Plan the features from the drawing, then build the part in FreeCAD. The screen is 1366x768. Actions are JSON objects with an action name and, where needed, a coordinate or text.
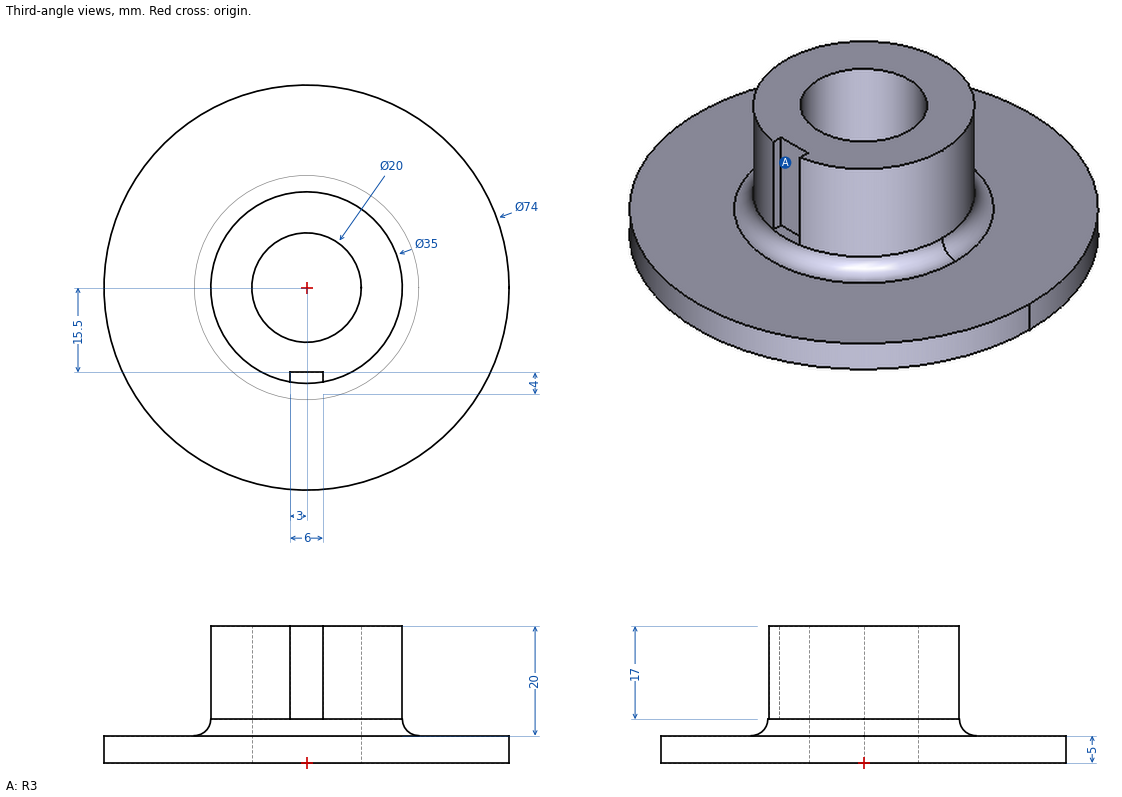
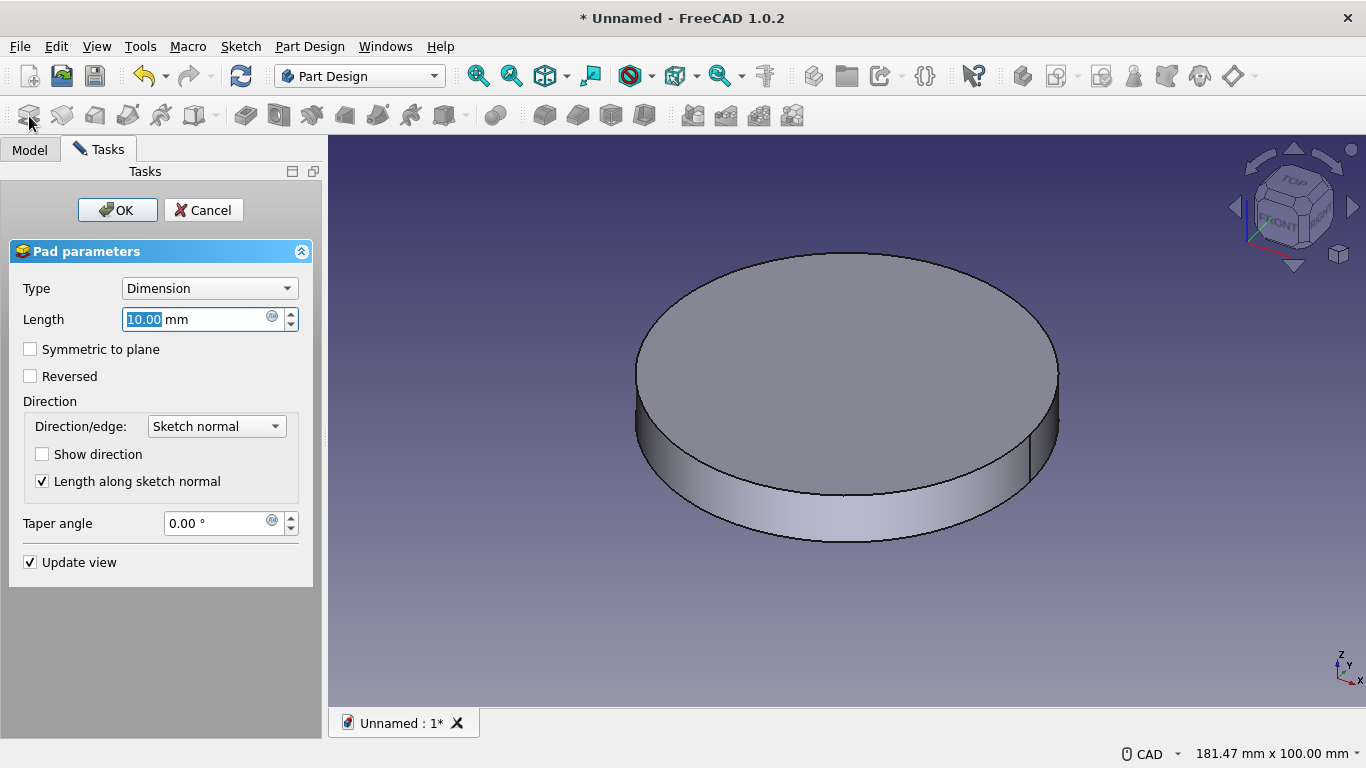
{"action": "type", "text": "5"}
{"action": "key", "text": "Tab"}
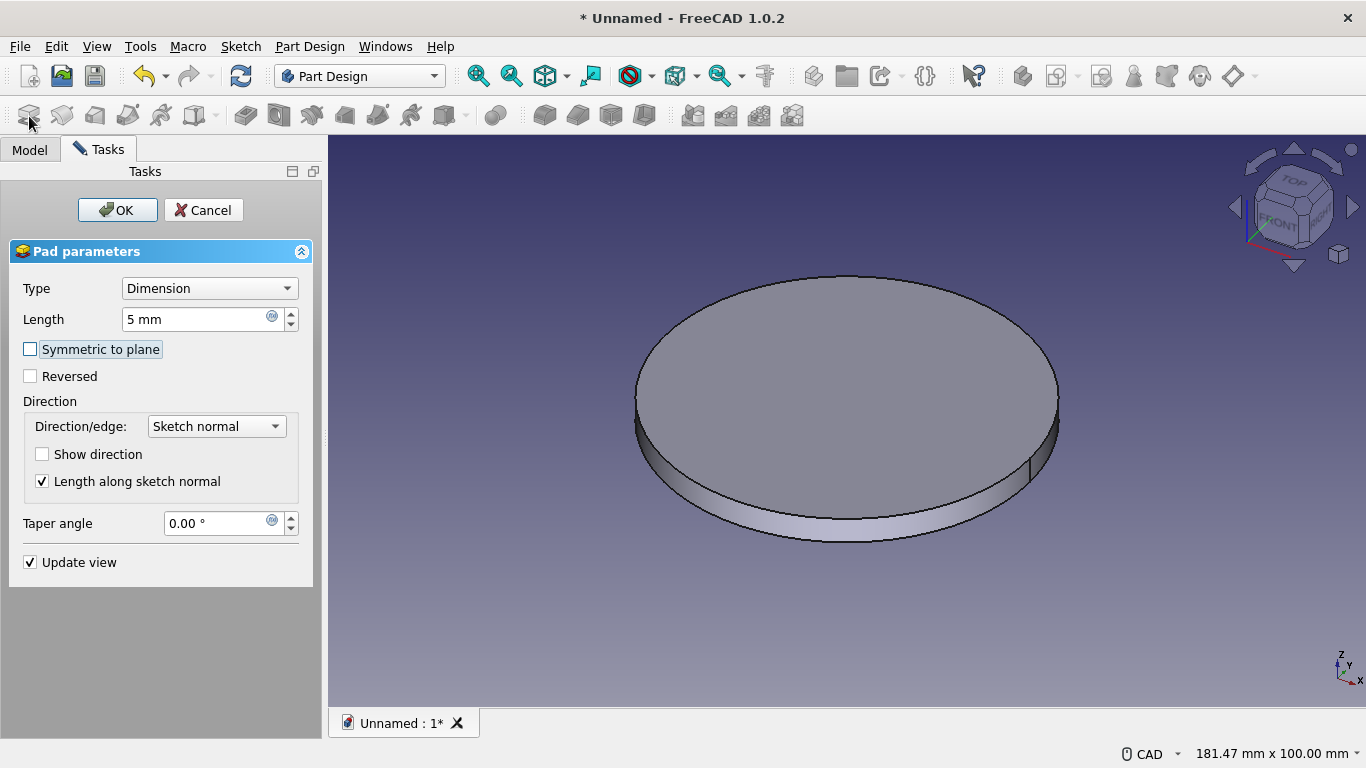
{"action": "left_click", "coordinate": [118, 210]}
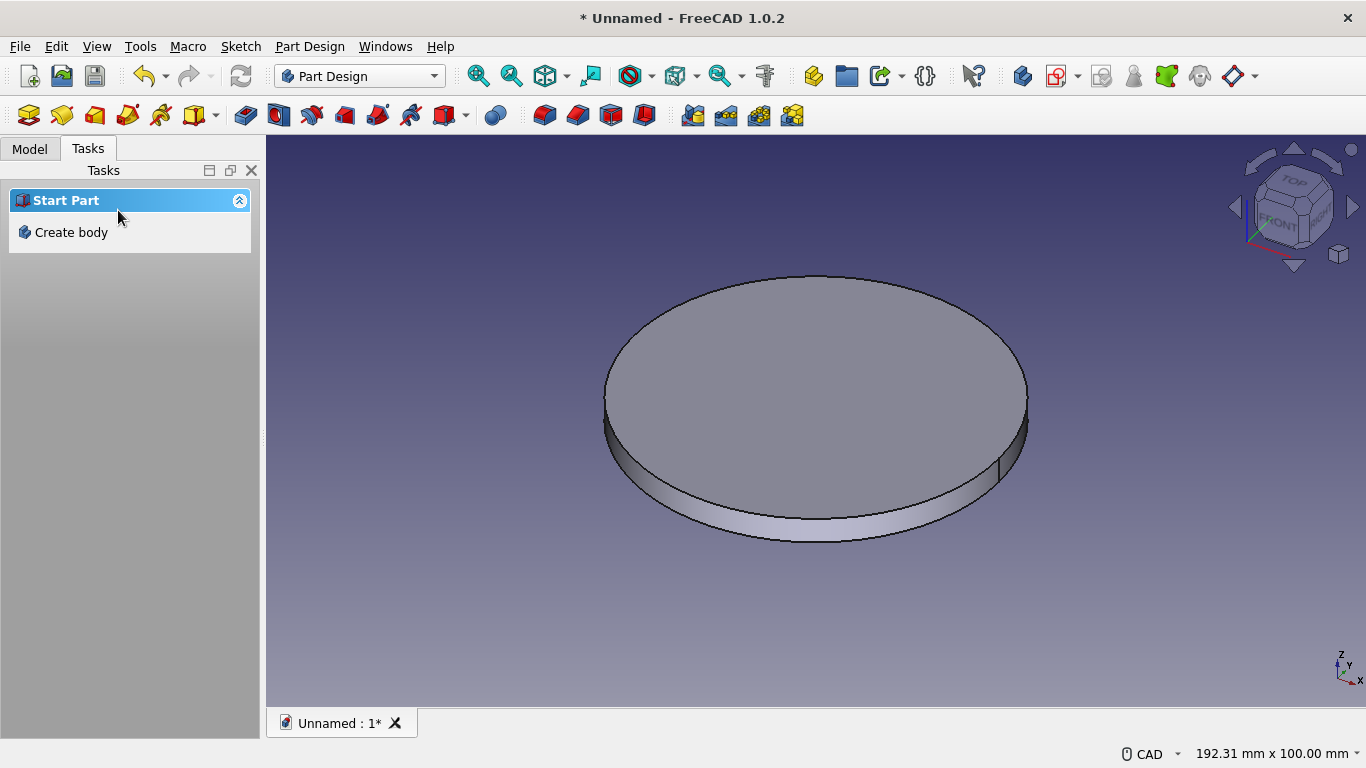
{"action": "left_click", "coordinate": [816, 397]}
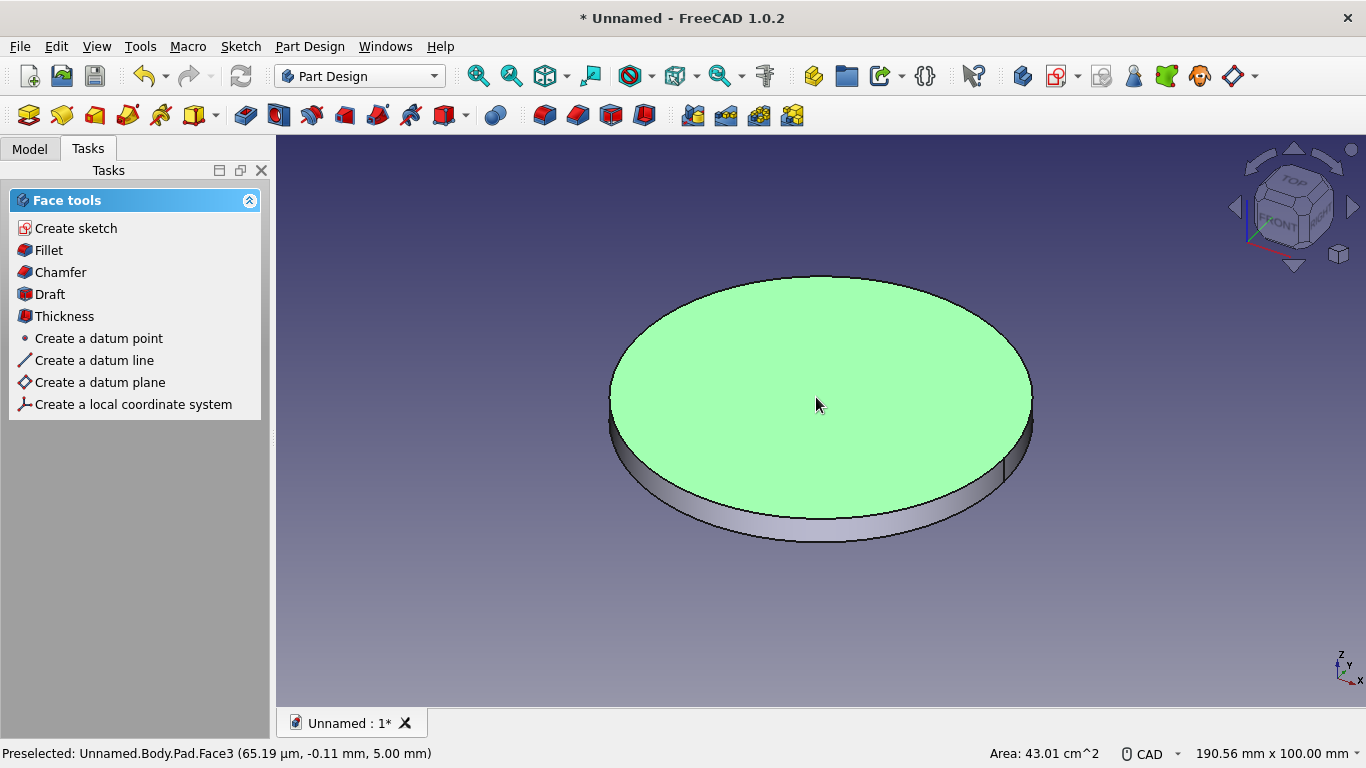
{"action": "left_click", "coordinate": [1056, 76]}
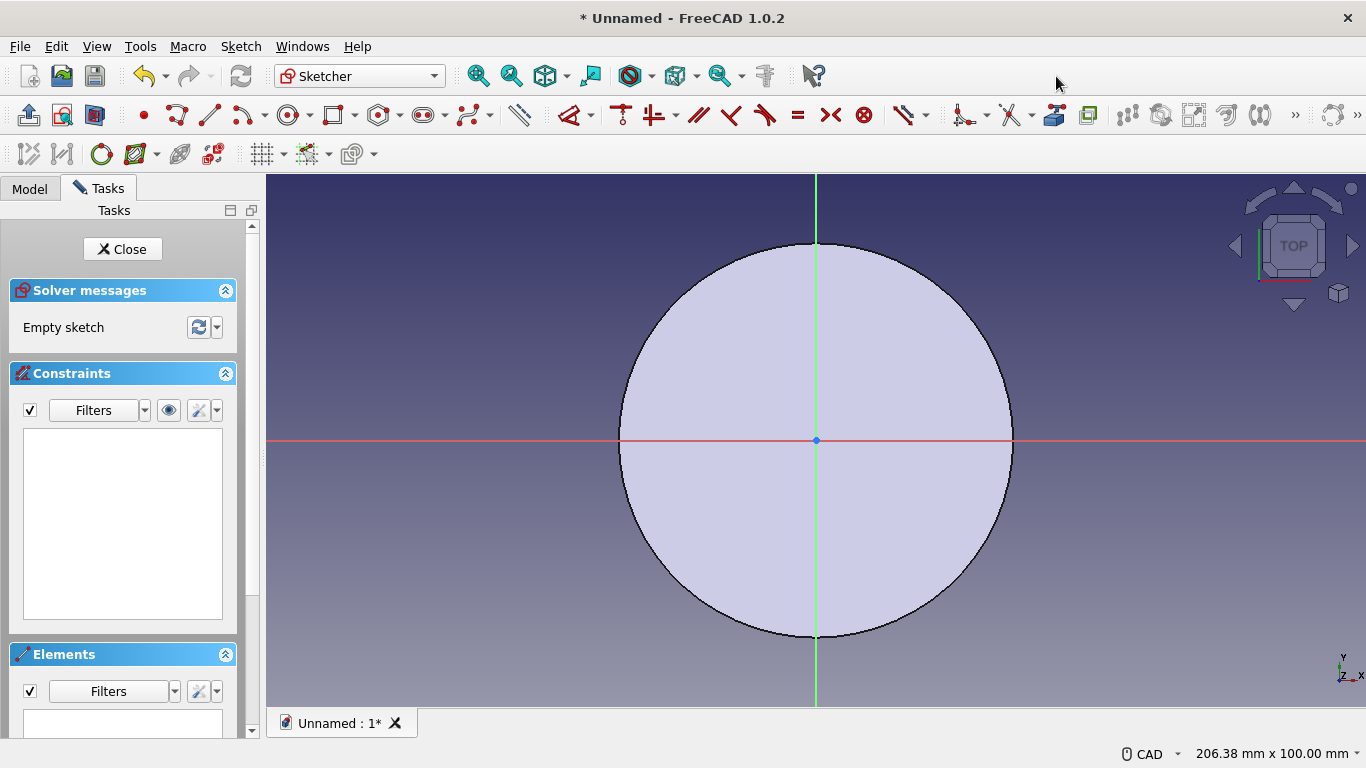
{"action": "scroll", "coordinate": [899, 441], "scroll_direction": "up", "scroll_amount": 3}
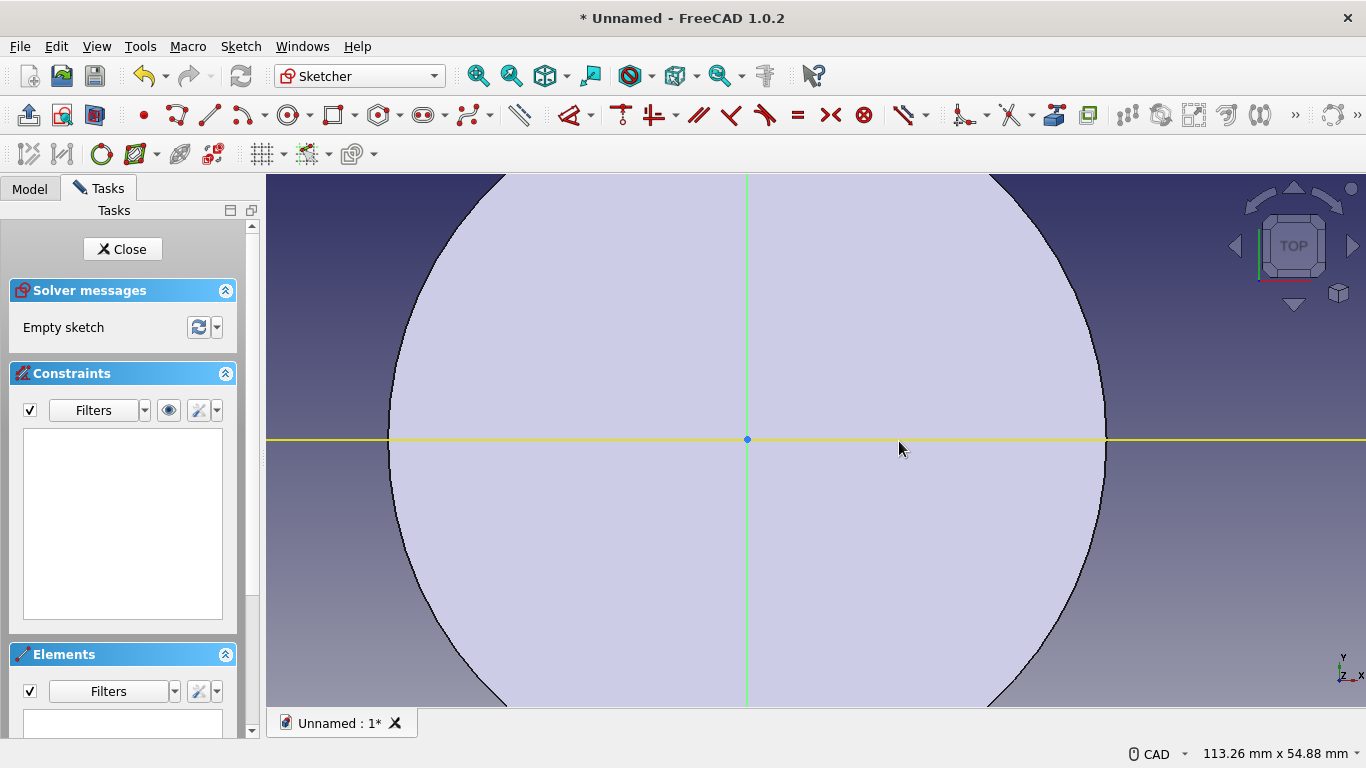
{"action": "left_click", "coordinate": [288, 116]}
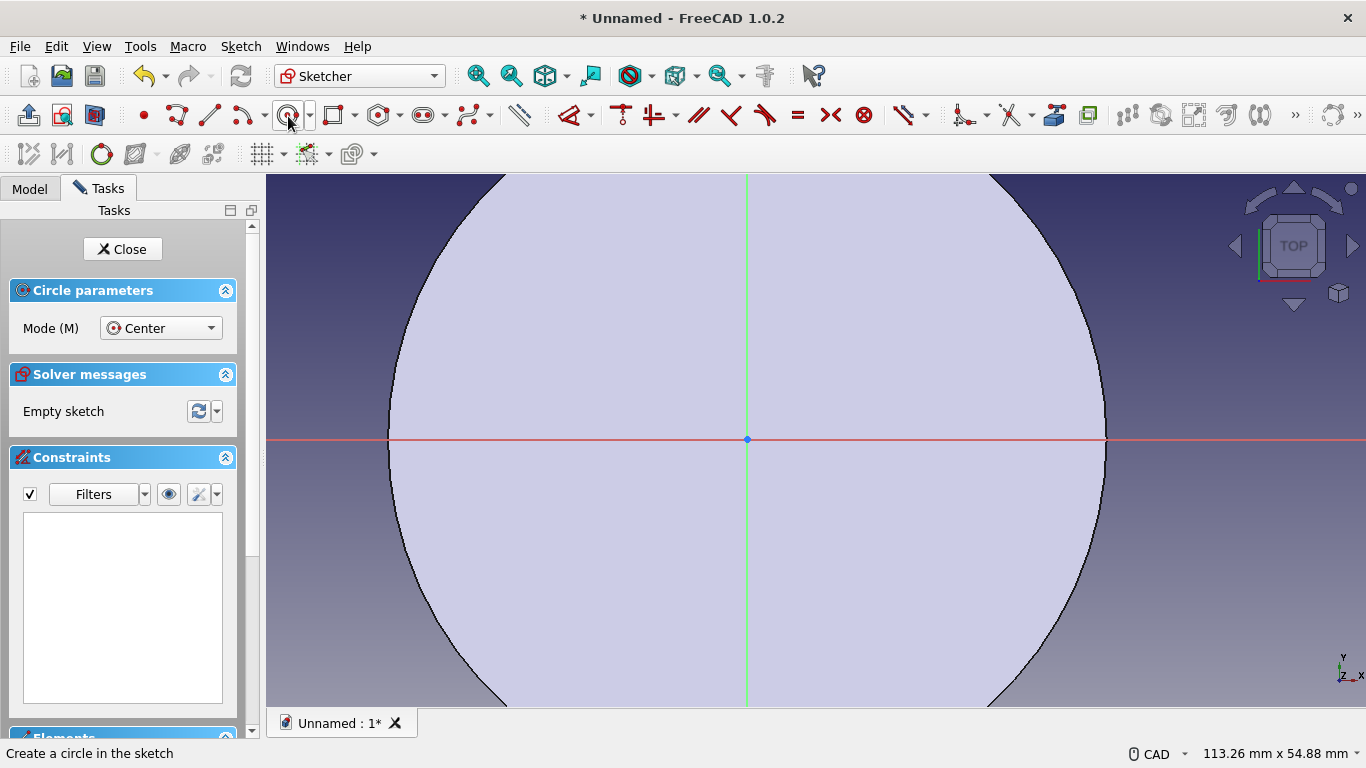
{"action": "left_click", "coordinate": [747, 440]}
{"action": "mouse_move", "coordinate": [867, 319]}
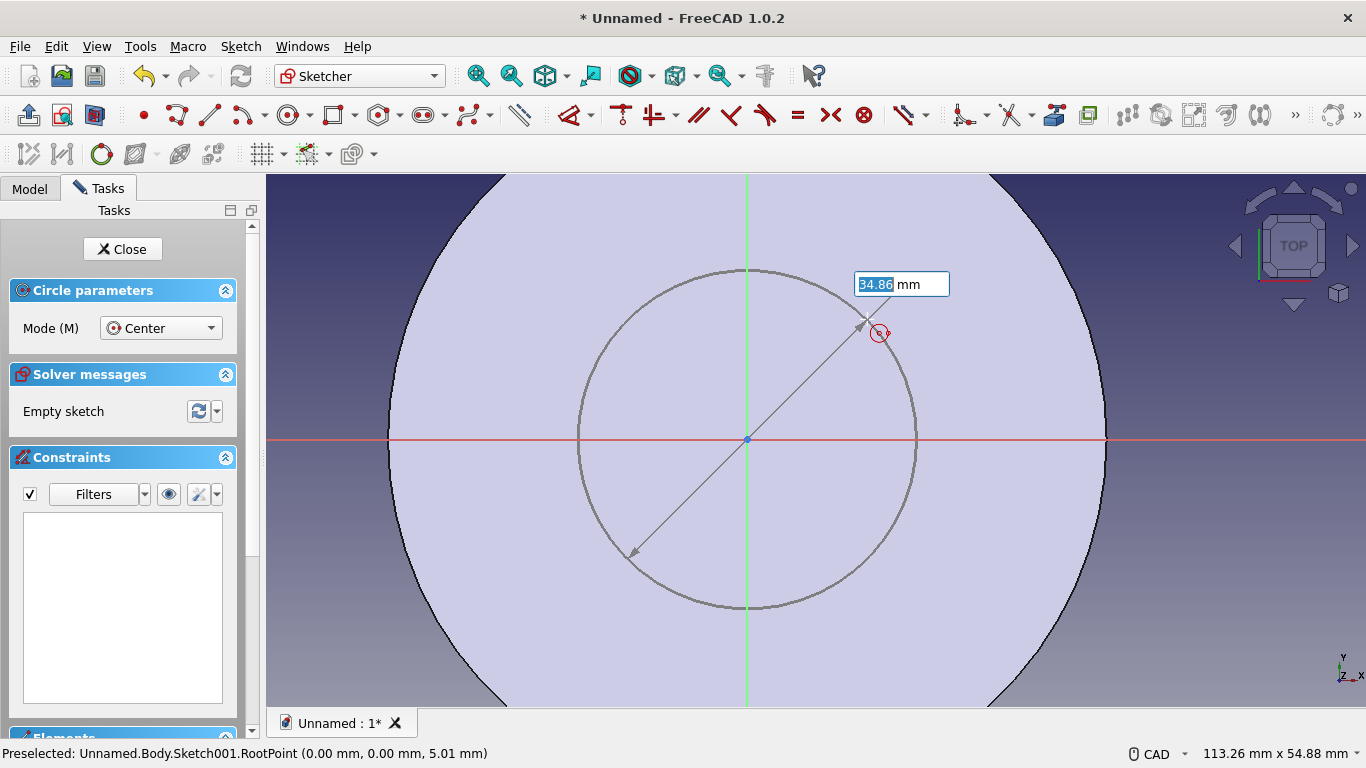
{"action": "type", "text": "35"}
{"action": "key", "text": "Return"}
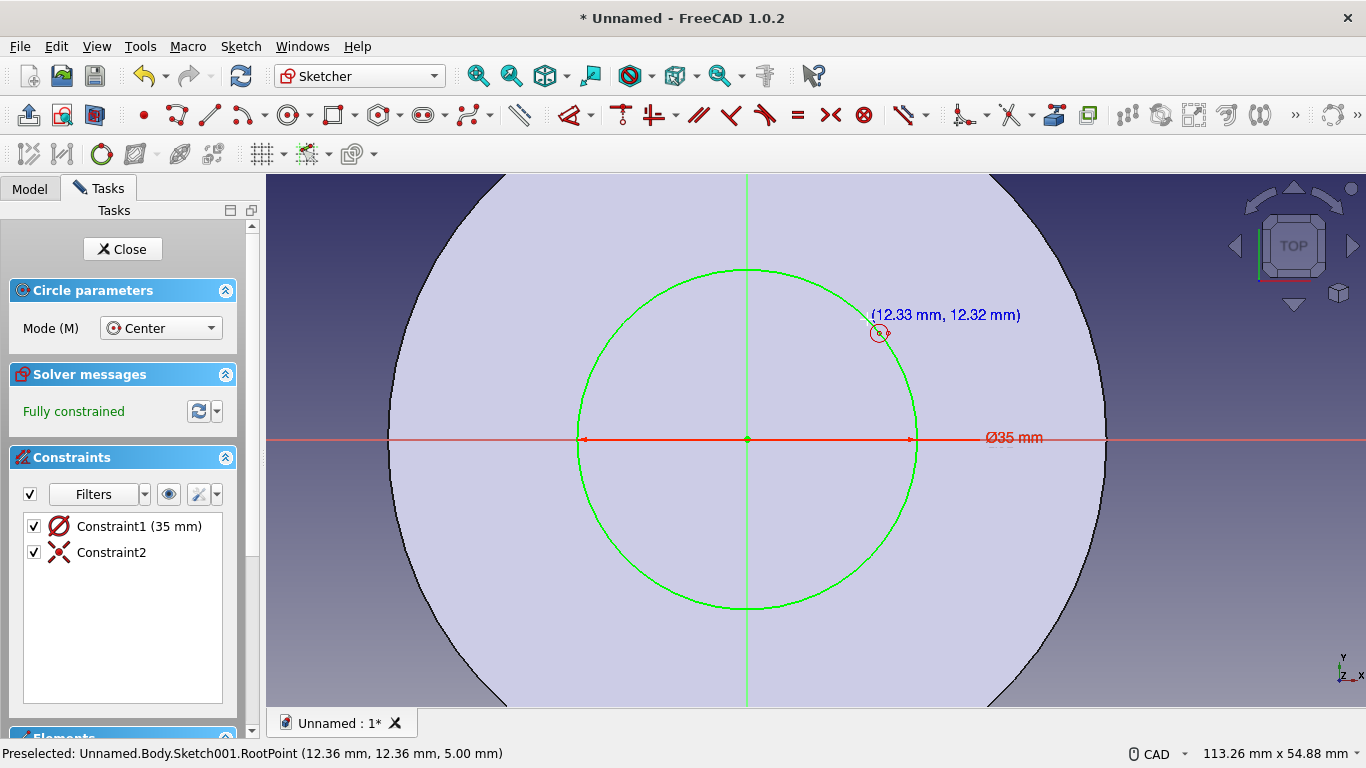
{"action": "left_click", "coordinate": [747, 440]}
{"action": "mouse_move", "coordinate": [816, 371]}